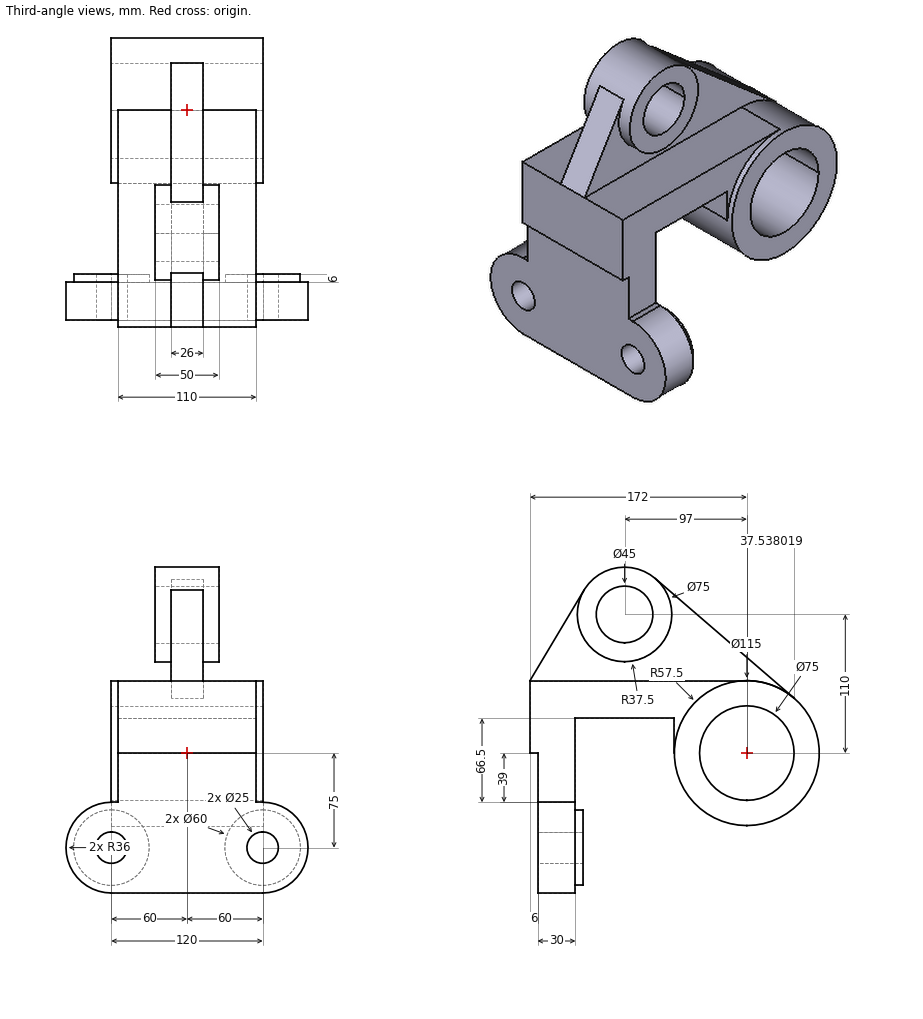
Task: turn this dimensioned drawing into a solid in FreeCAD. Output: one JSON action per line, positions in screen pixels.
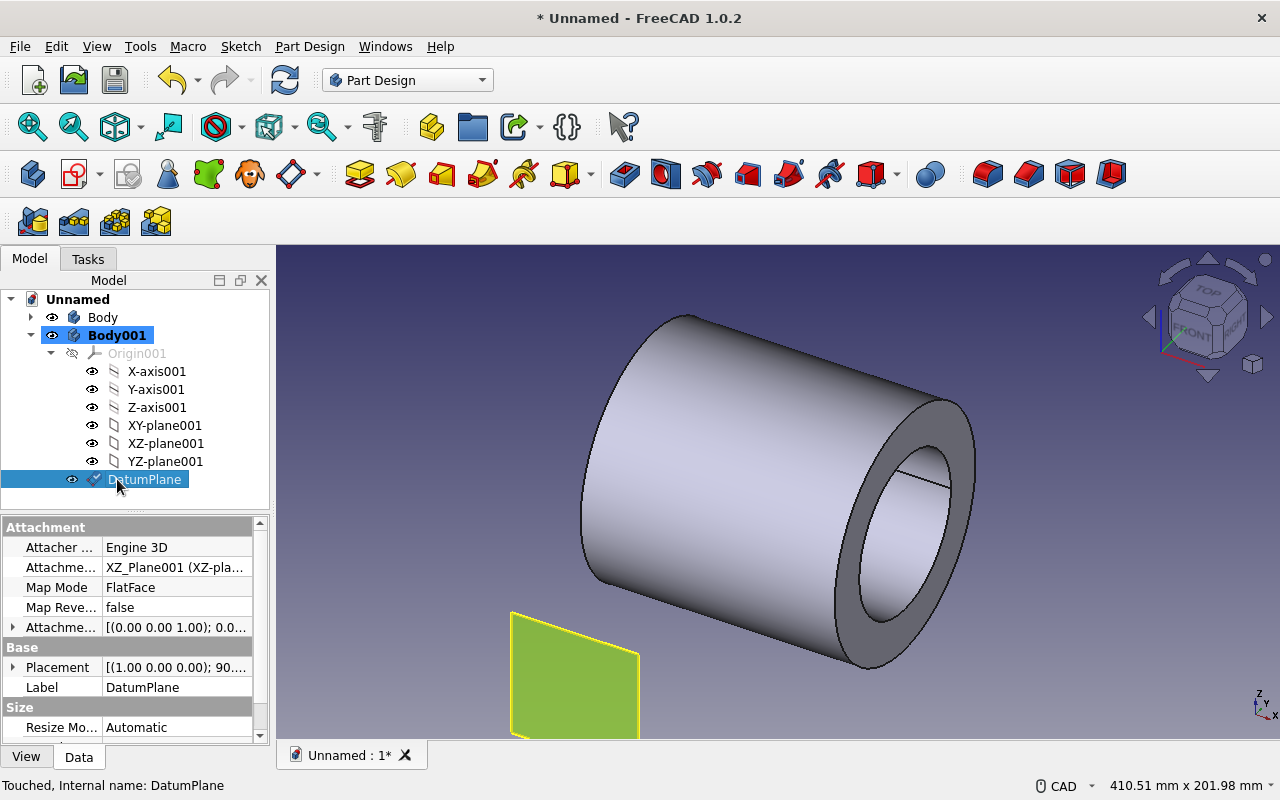
{"action": "left_click", "coordinate": [74, 174]}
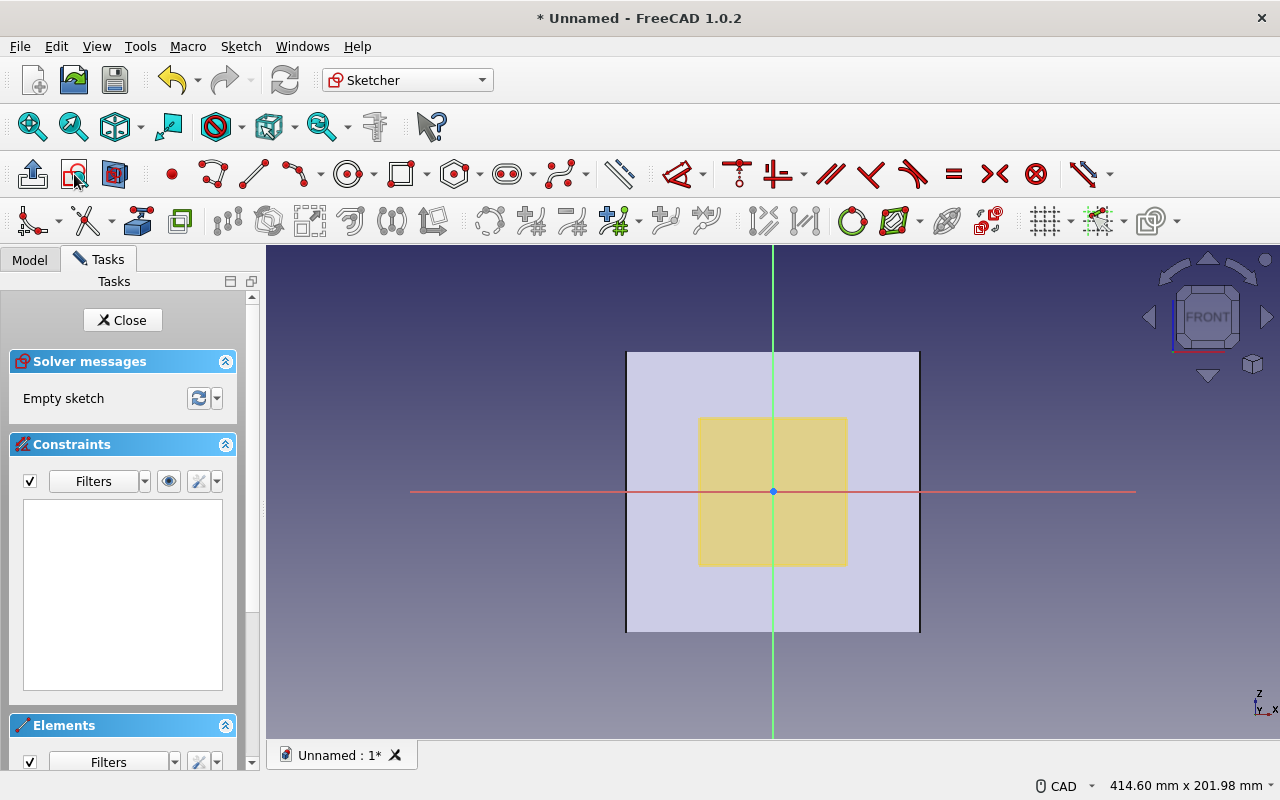
{"action": "scroll", "coordinate": [395, 273], "scroll_direction": "down", "scroll_amount": 1}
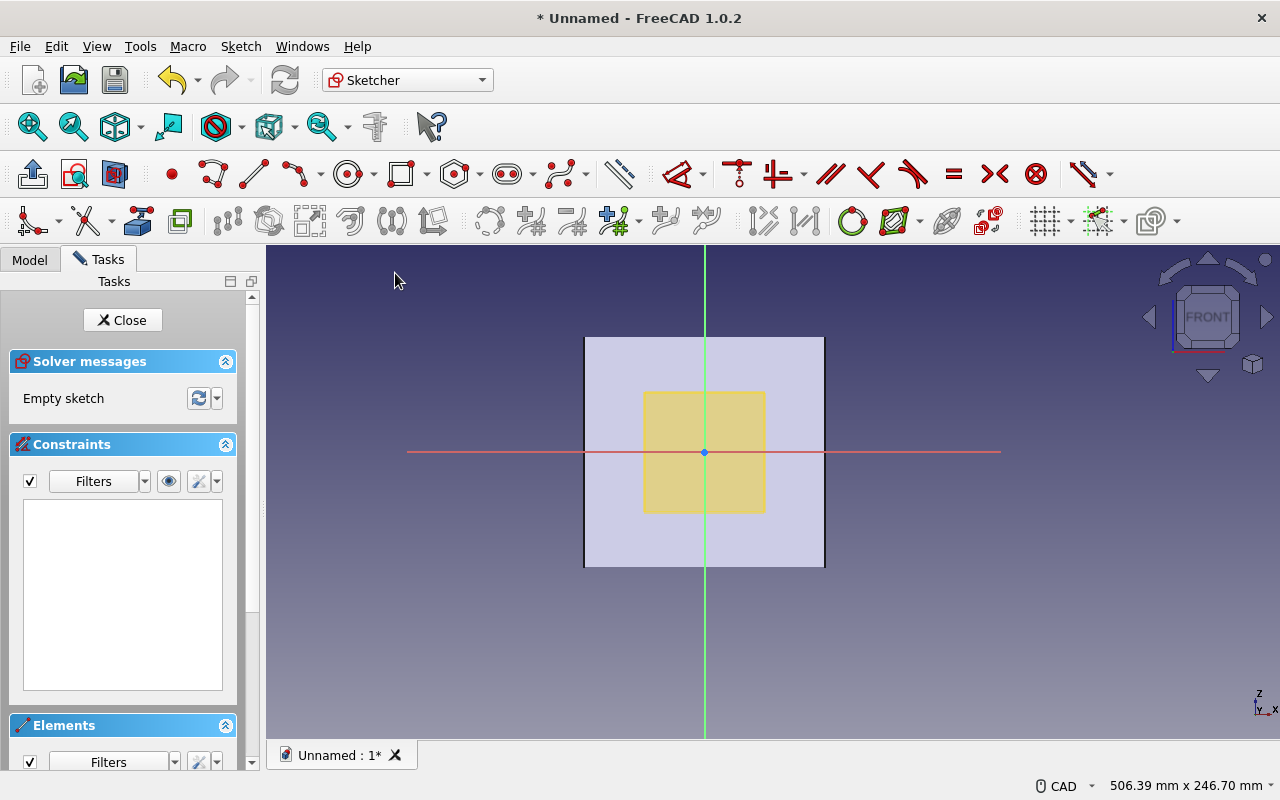
{"action": "scroll", "coordinate": [705, 709], "scroll_direction": "up", "scroll_amount": 2}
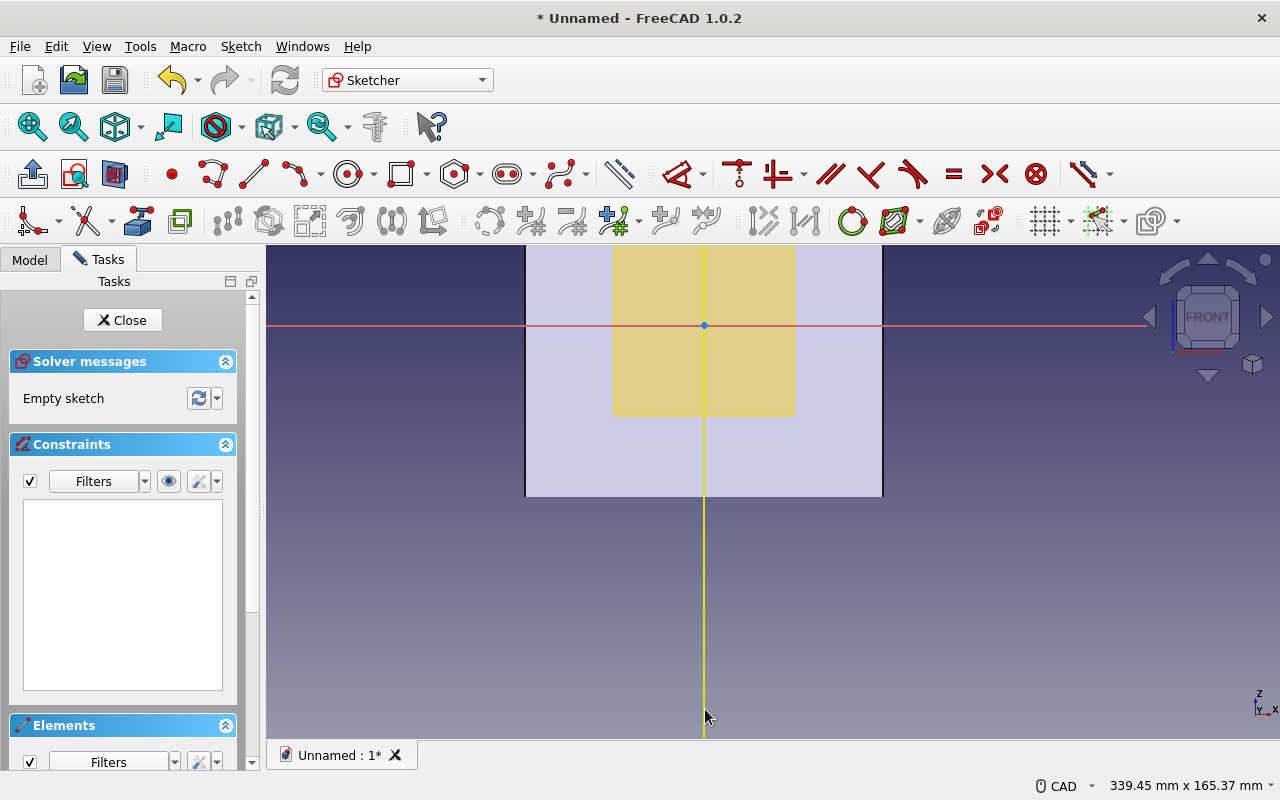
{"action": "key", "text": "g s"}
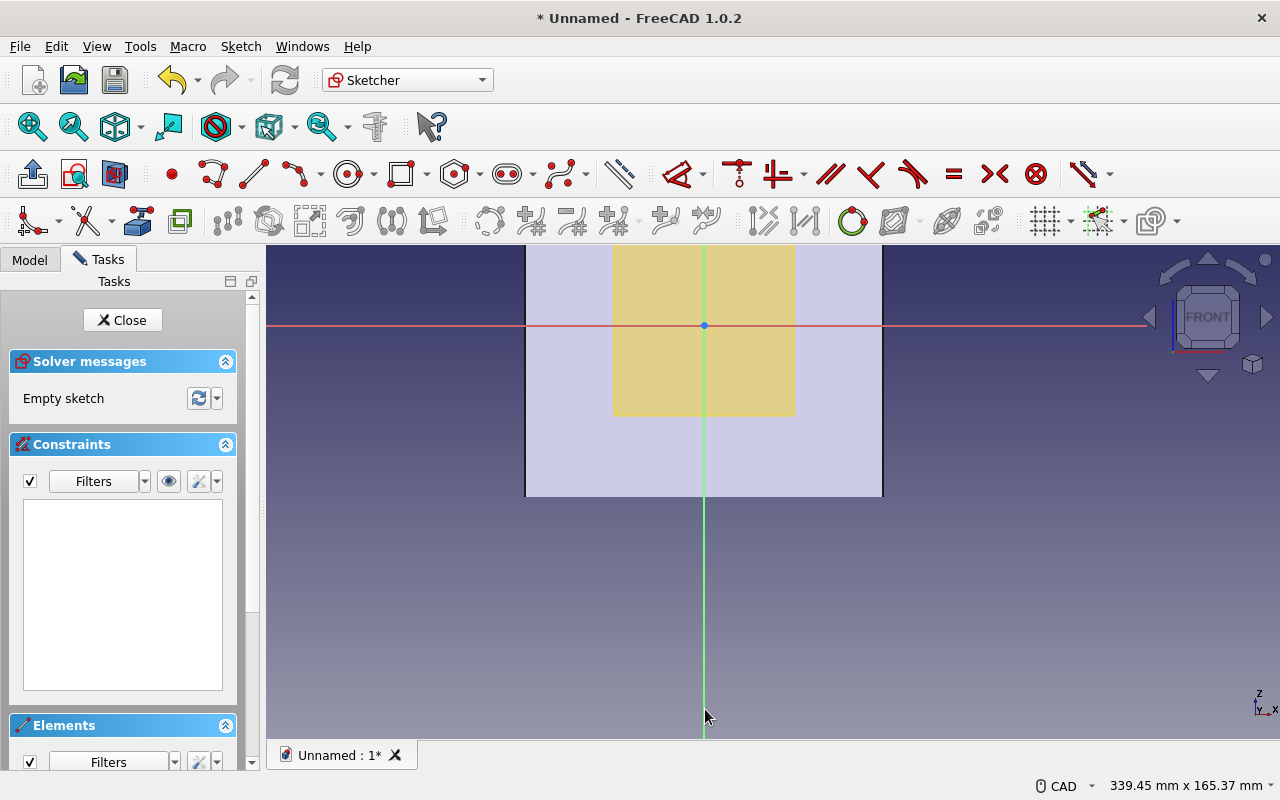
{"action": "left_click", "coordinate": [525, 550]}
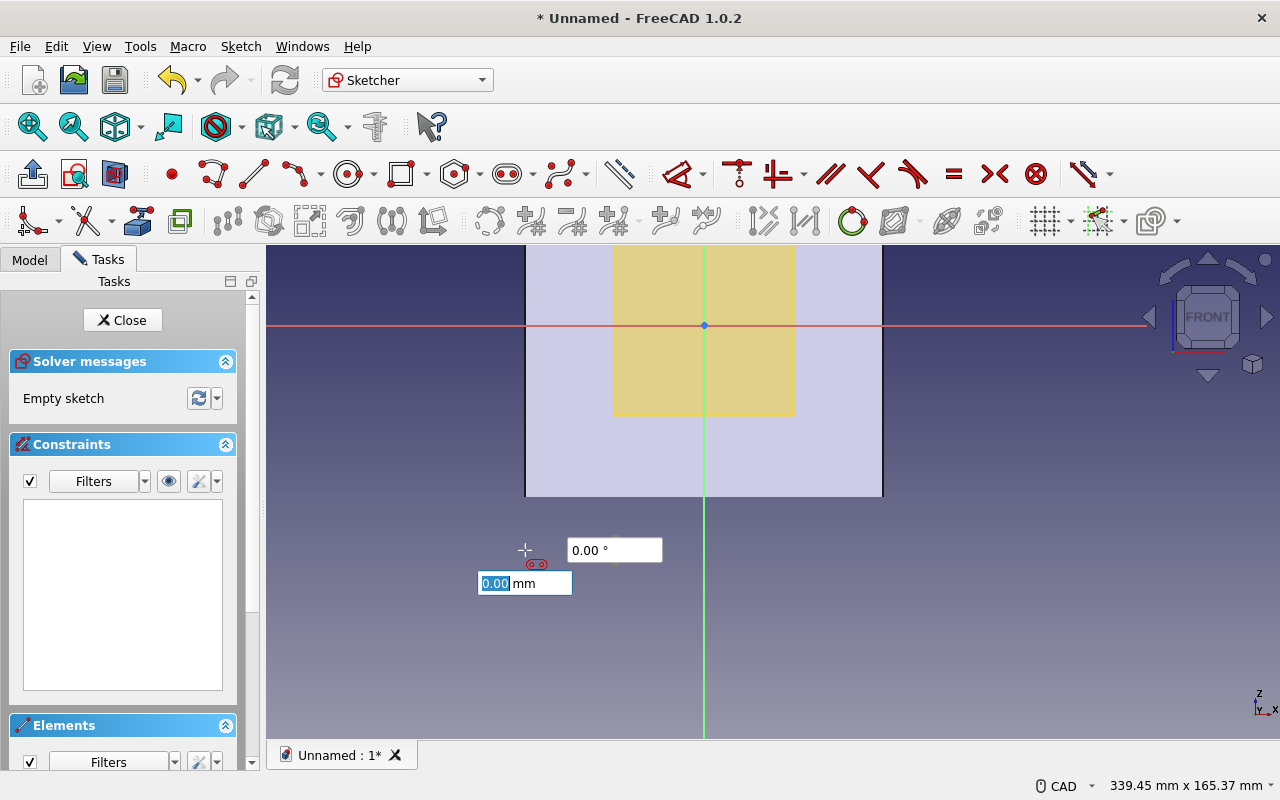
{"action": "left_click", "coordinate": [883, 550]}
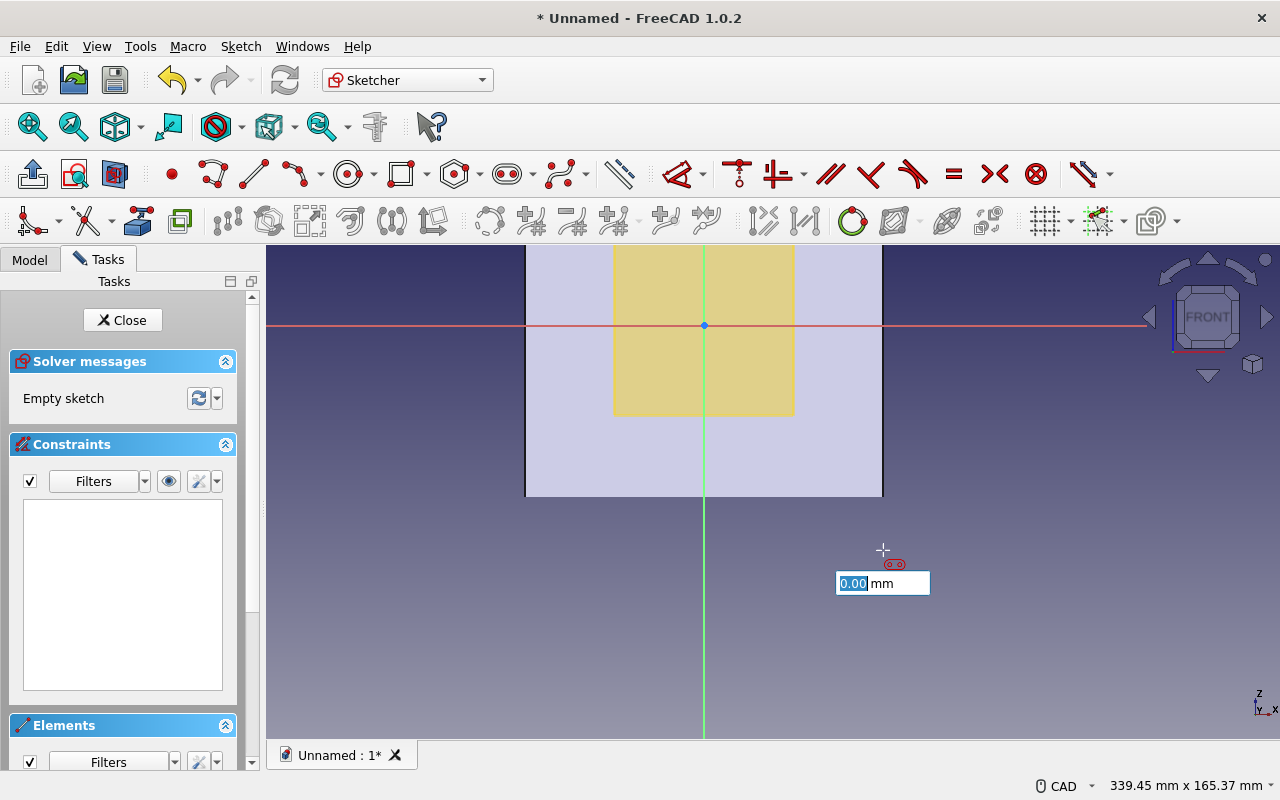
{"action": "left_click", "coordinate": [758, 657]}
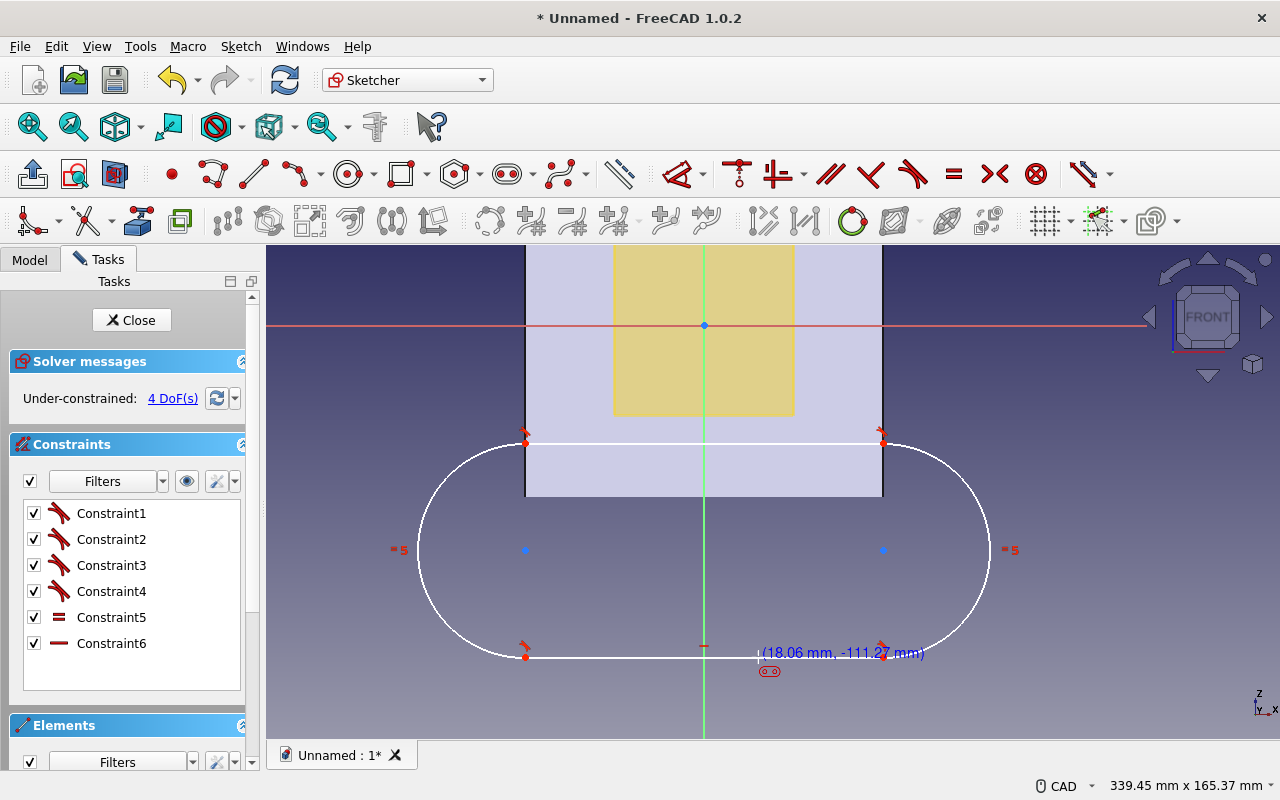
{"action": "key", "text": "g c"}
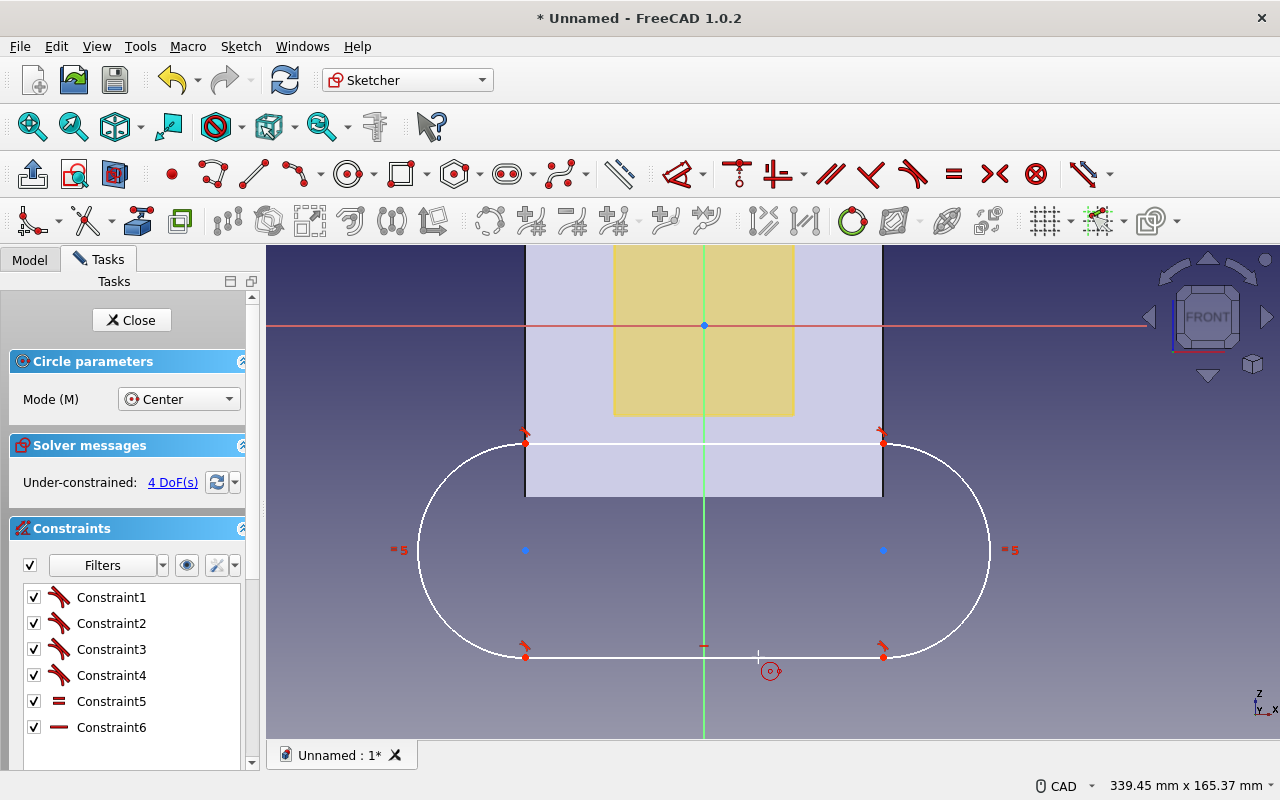
{"action": "left_click", "coordinate": [883, 551]}
{"action": "left_click", "coordinate": [910, 523]}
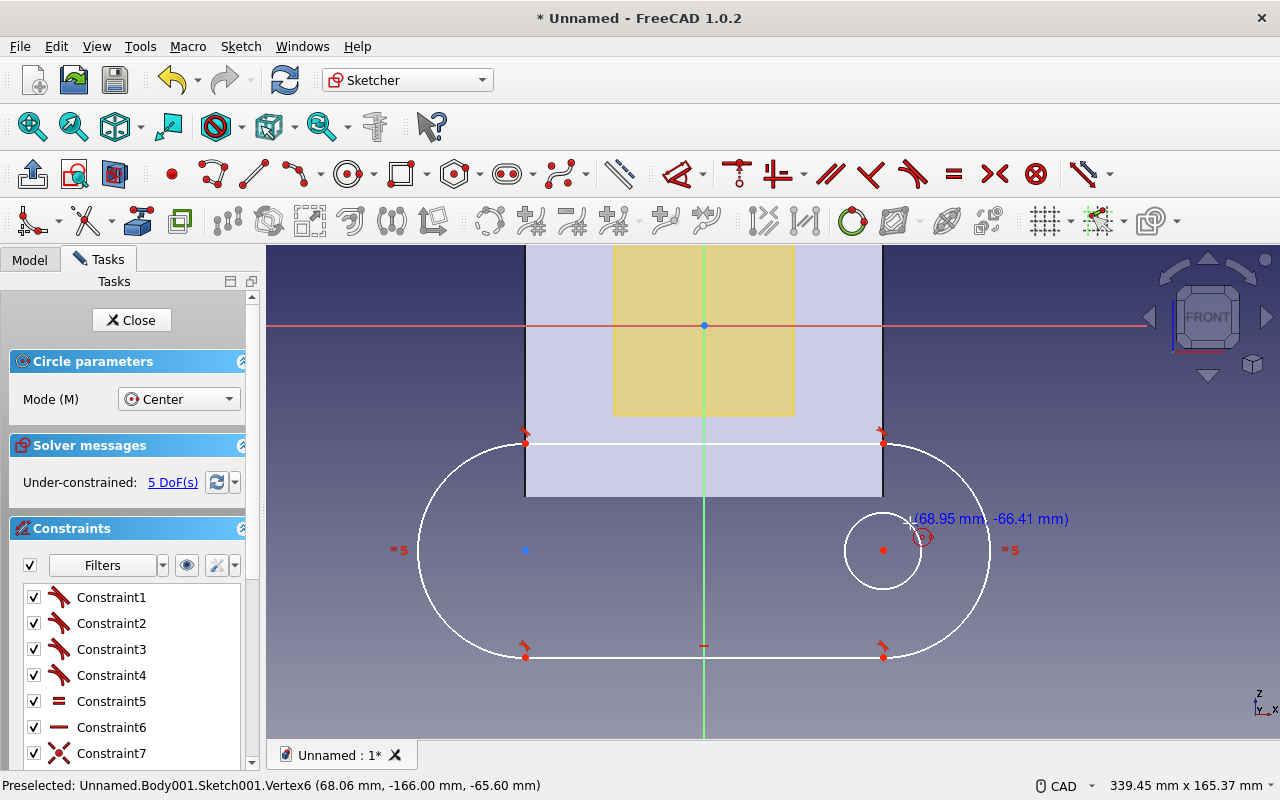
{"action": "left_click", "coordinate": [525, 551]}
{"action": "left_click", "coordinate": [551, 523]}
{"action": "key", "text": "Escape"}